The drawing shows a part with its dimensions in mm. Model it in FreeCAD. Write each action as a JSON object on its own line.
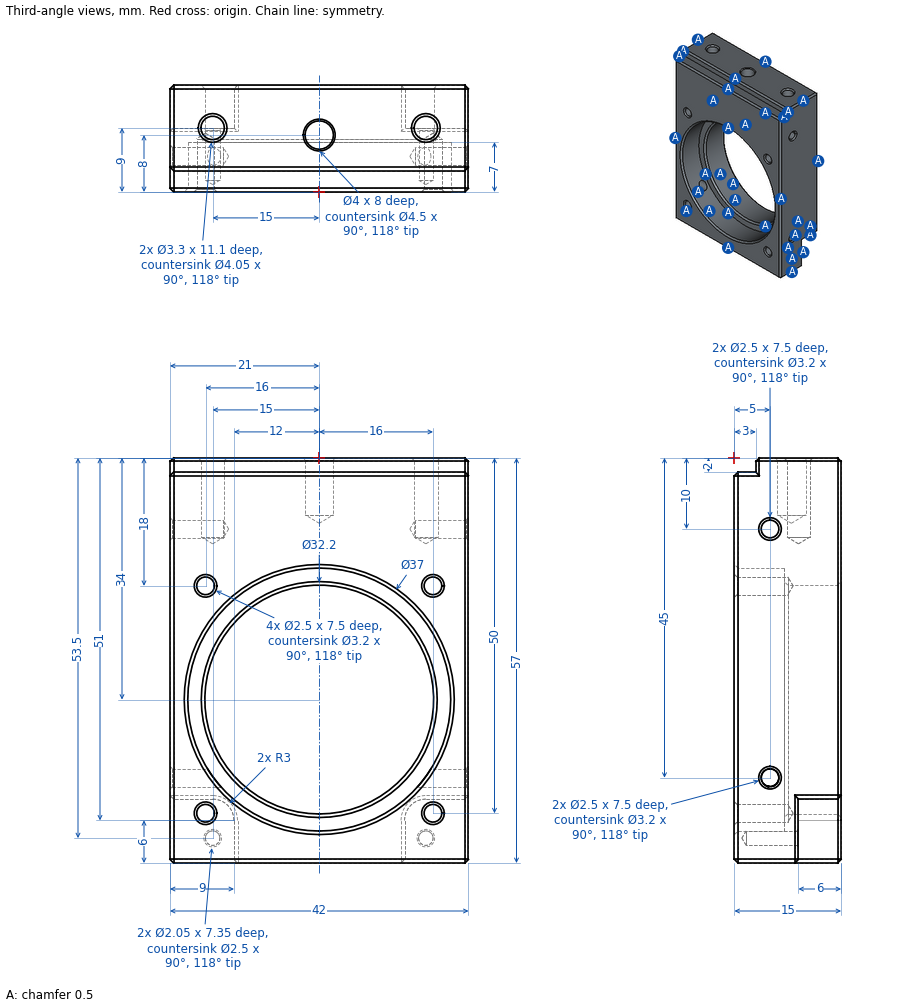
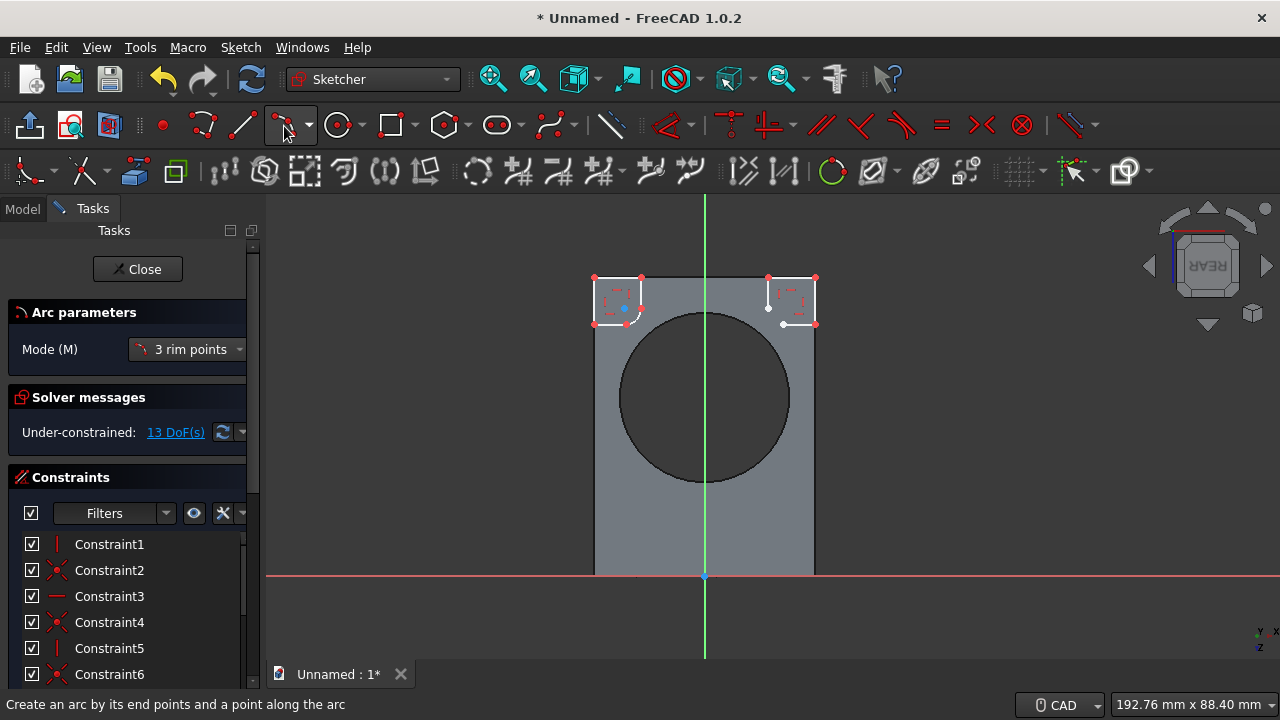
{"action": "left_click", "coordinate": [768, 309]}
{"action": "left_click", "coordinate": [783, 325]}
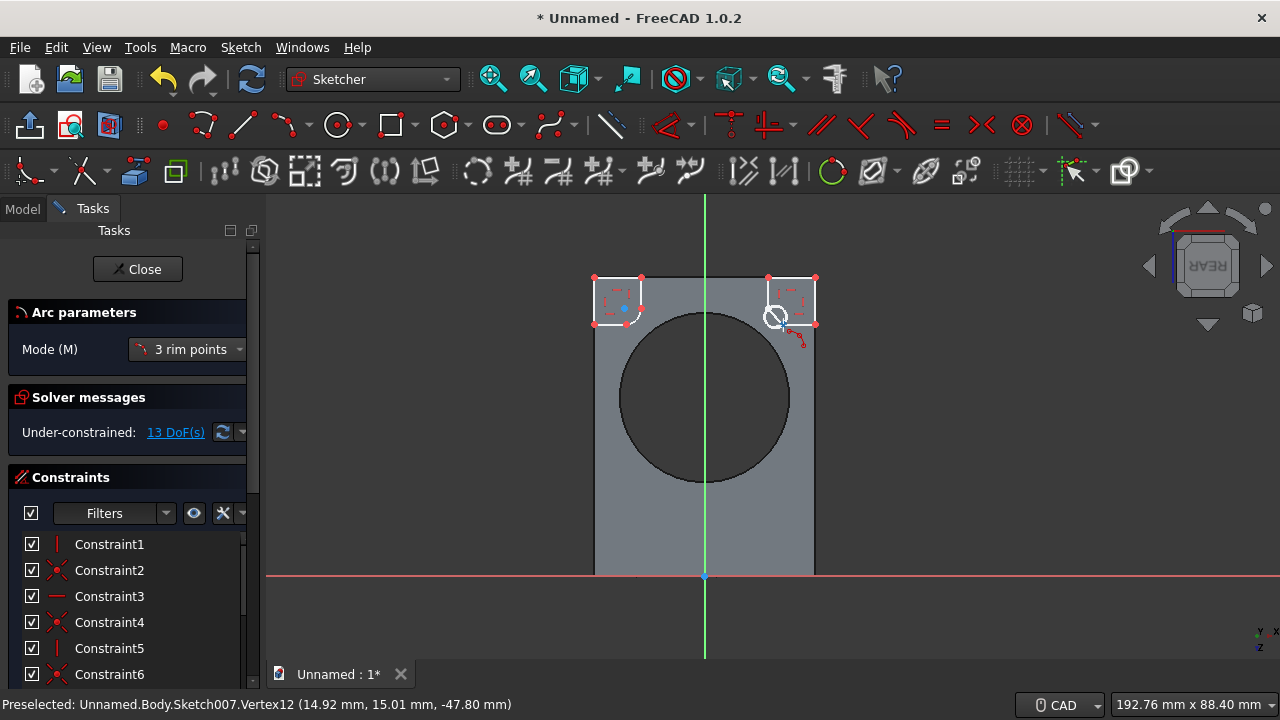
{"action": "scroll", "coordinate": [772, 319], "scroll_direction": "up", "scroll_amount": 7}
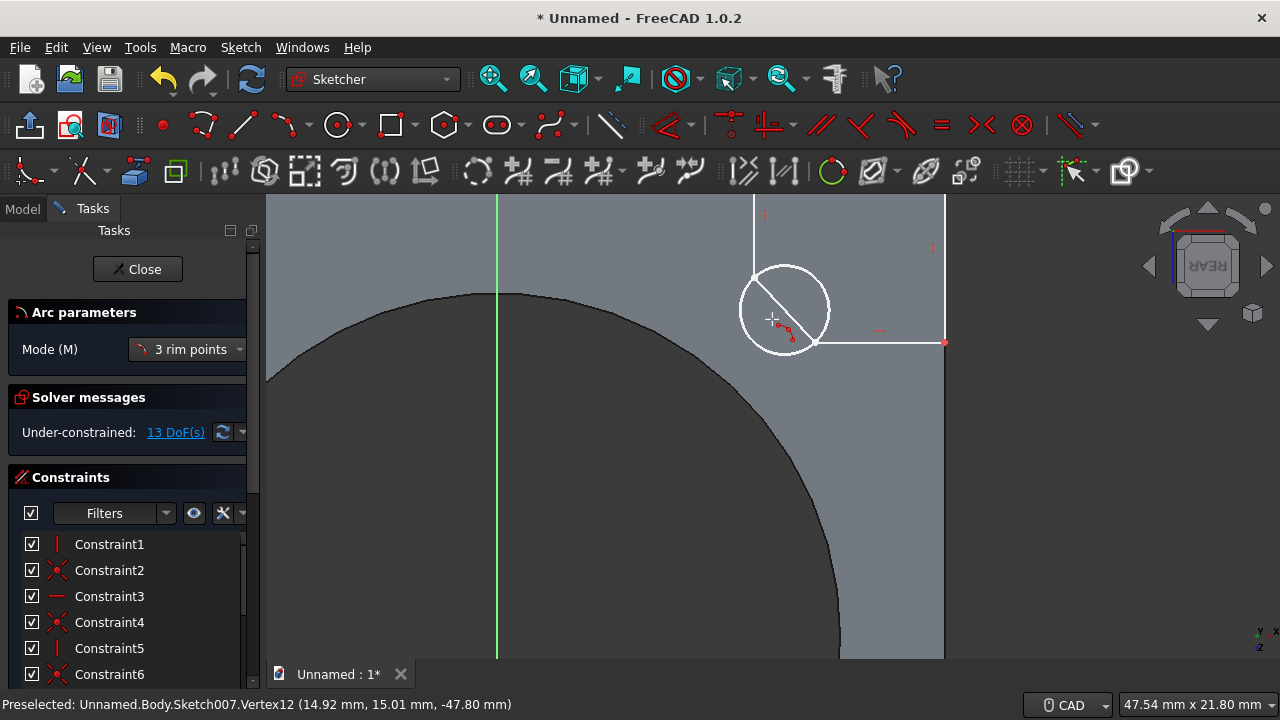
{"action": "left_click", "coordinate": [771, 319]}
{"action": "key", "text": "Escape"}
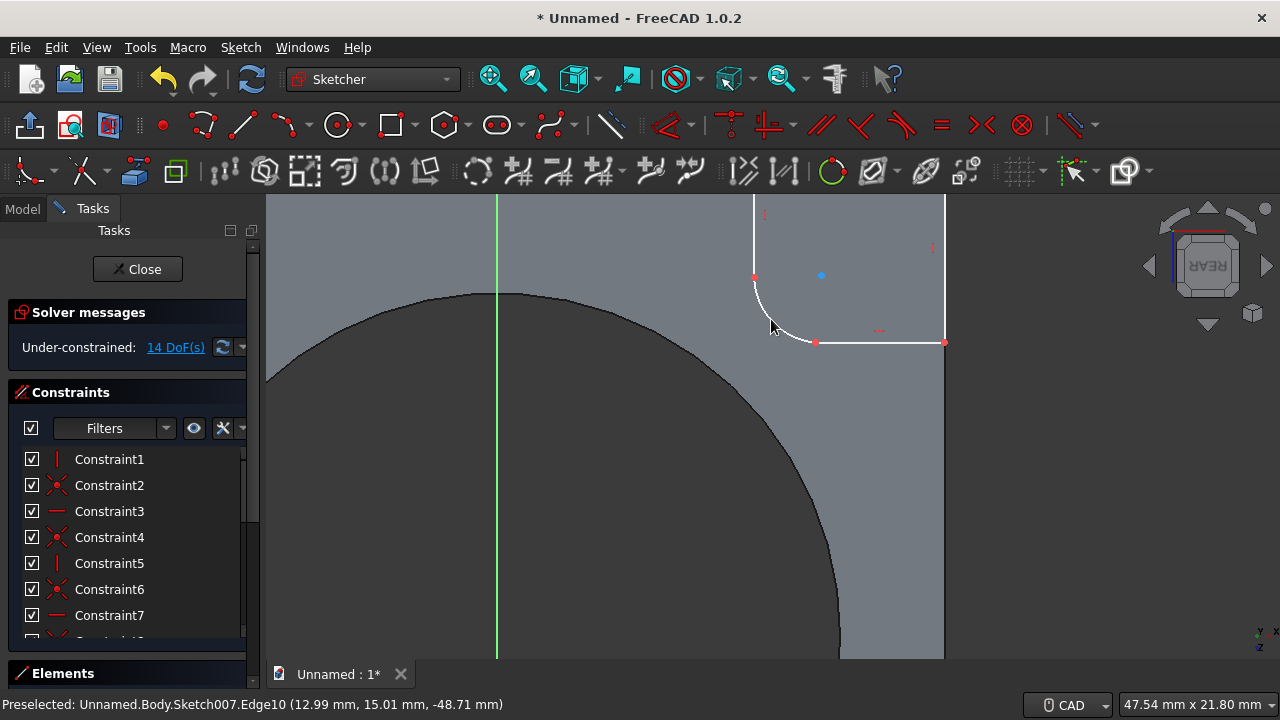
{"action": "scroll", "coordinate": [772, 319], "scroll_direction": "down", "scroll_amount": 7}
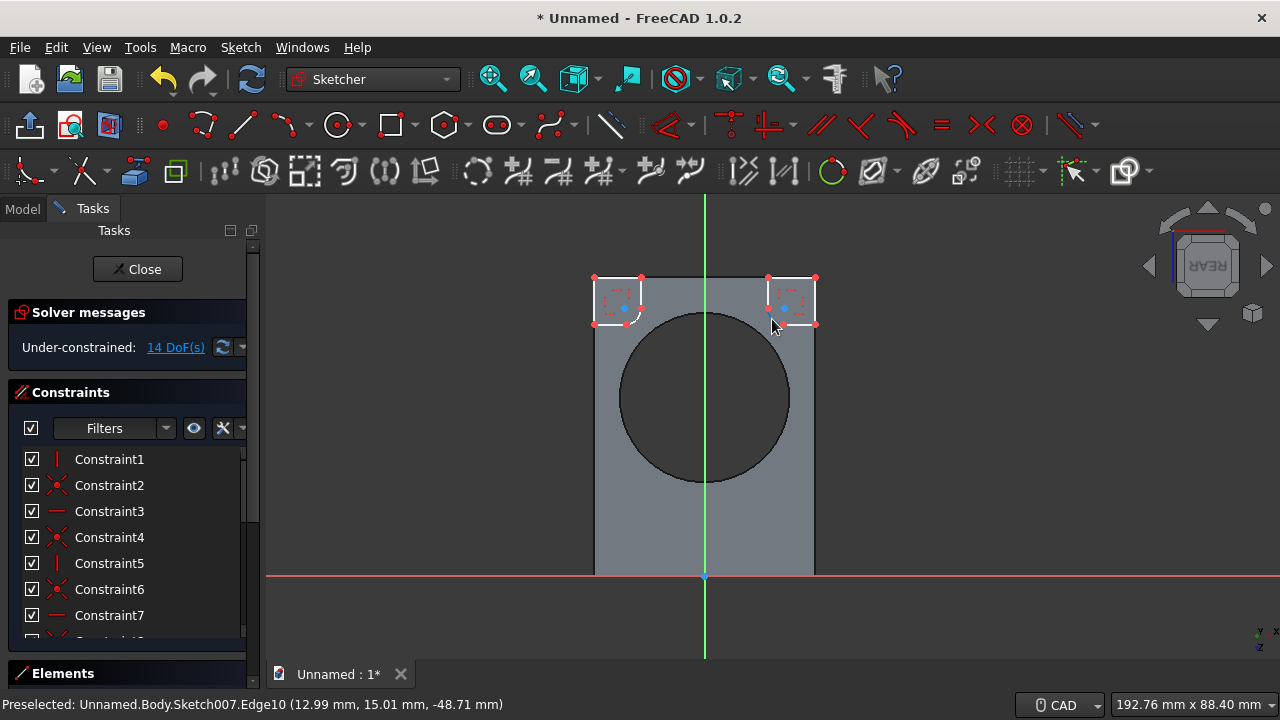
{"action": "scroll", "coordinate": [641, 300], "scroll_direction": "up", "scroll_amount": 2}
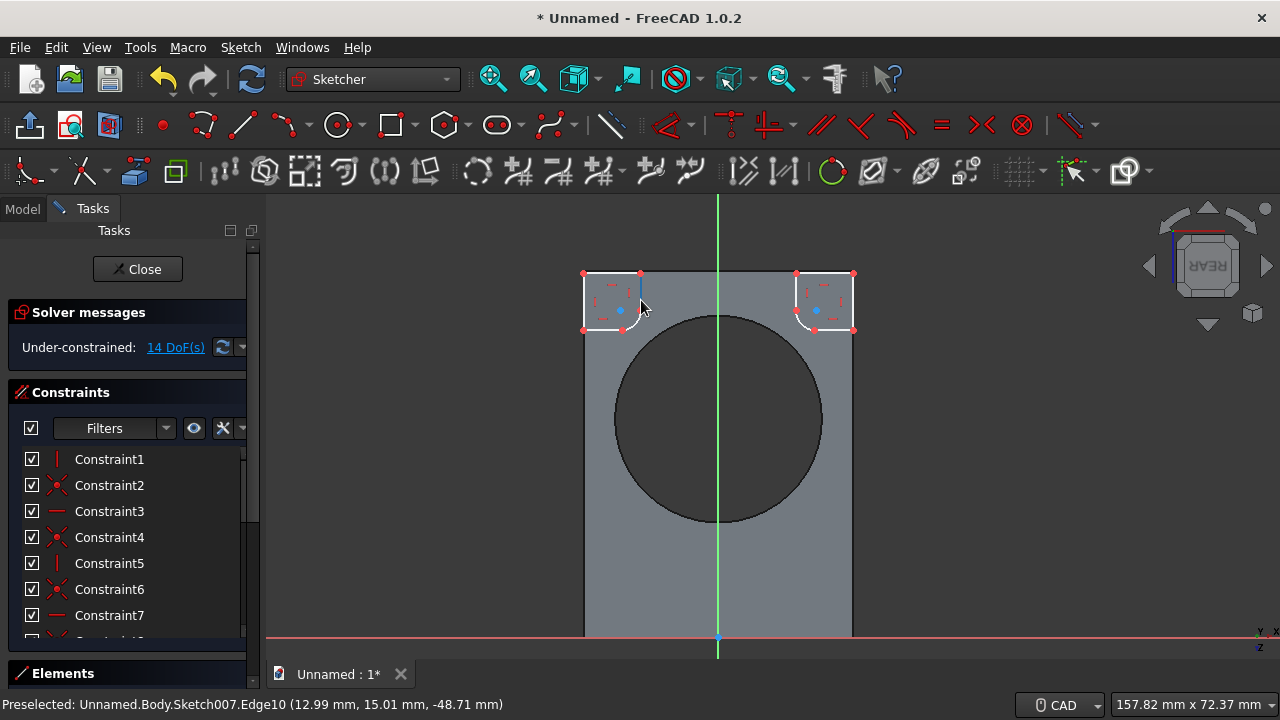
{"action": "left_click", "coordinate": [641, 299]}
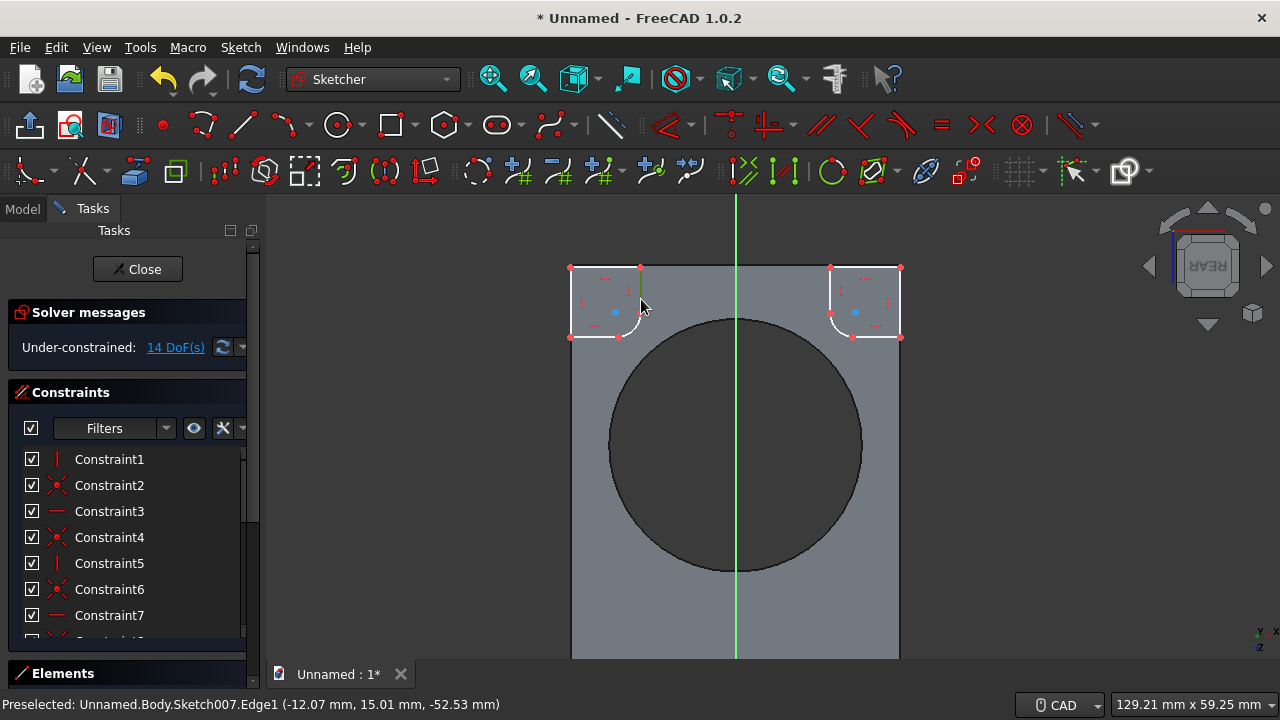
{"action": "scroll", "coordinate": [629, 334], "scroll_direction": "up", "scroll_amount": 2}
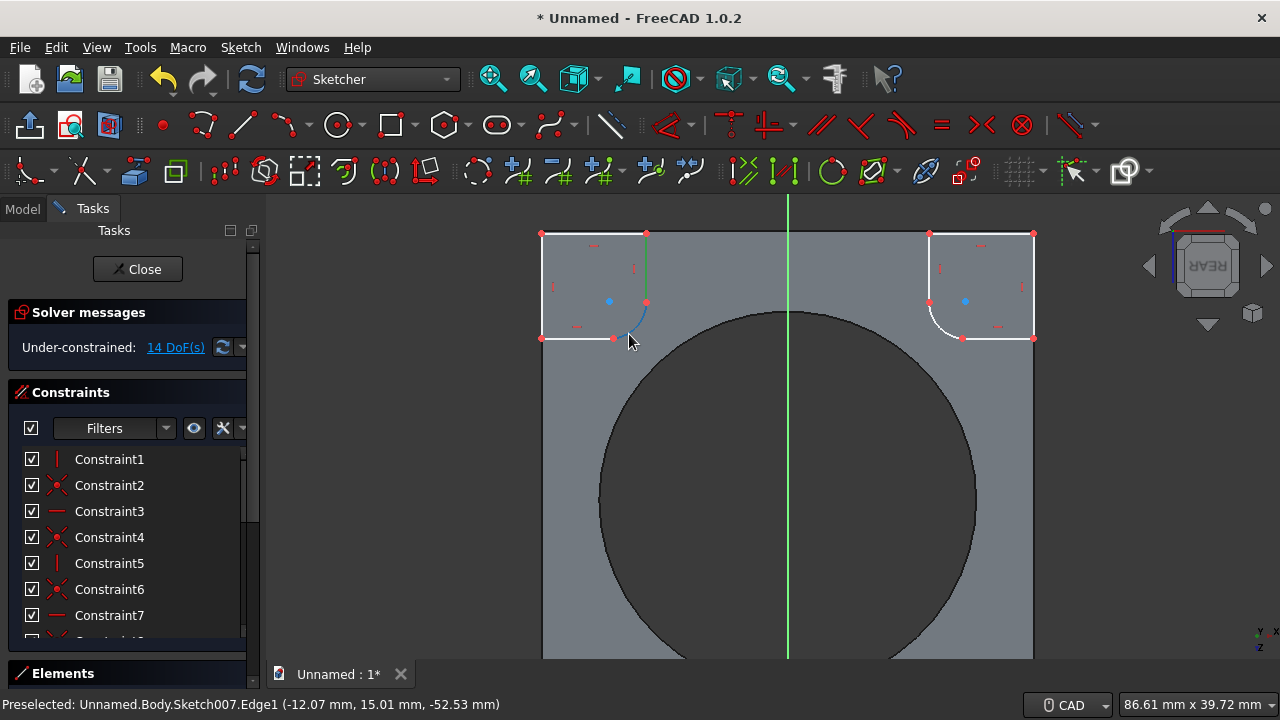
{"action": "left_click", "coordinate": [628, 334]}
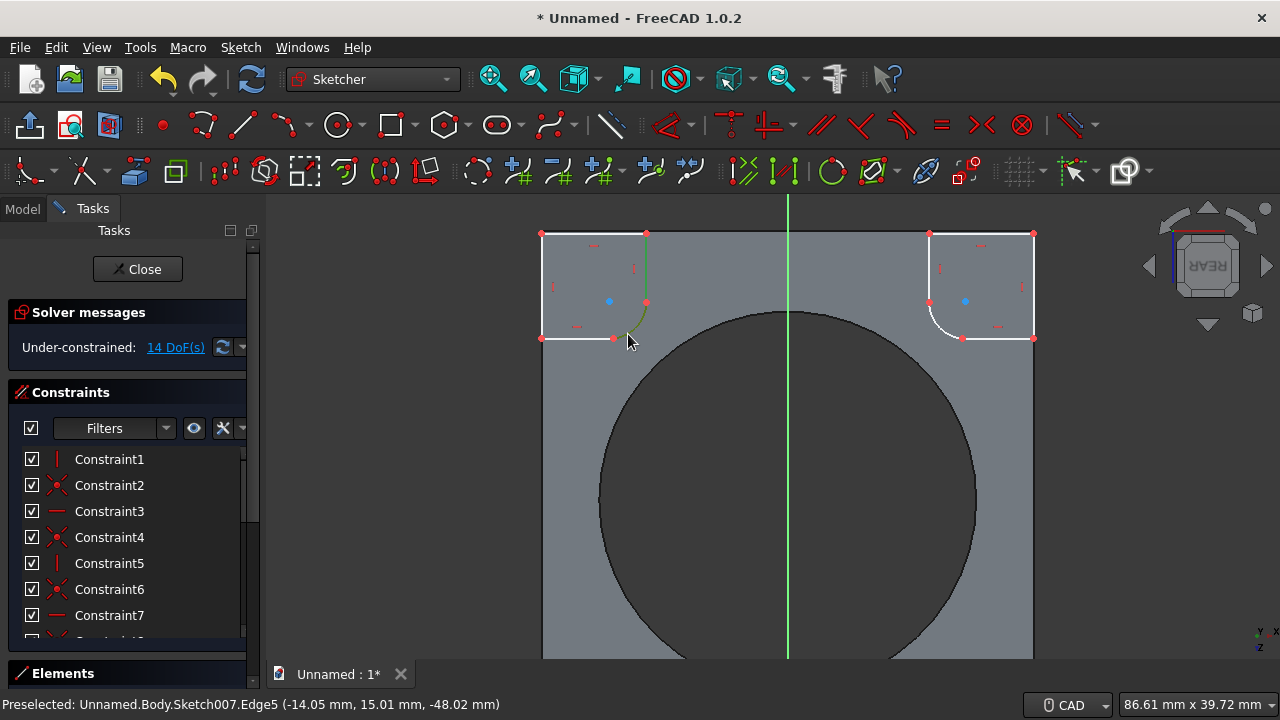
{"action": "key", "text": "t"}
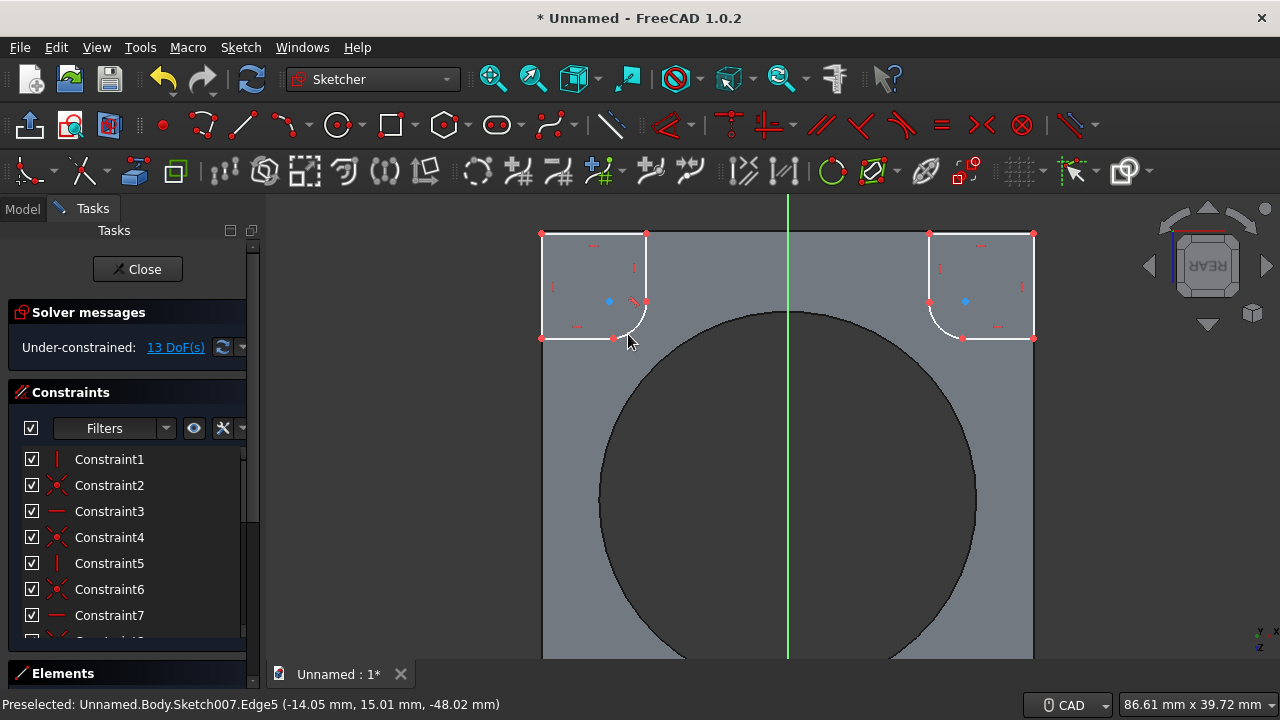
{"action": "left_click", "coordinate": [563, 339]}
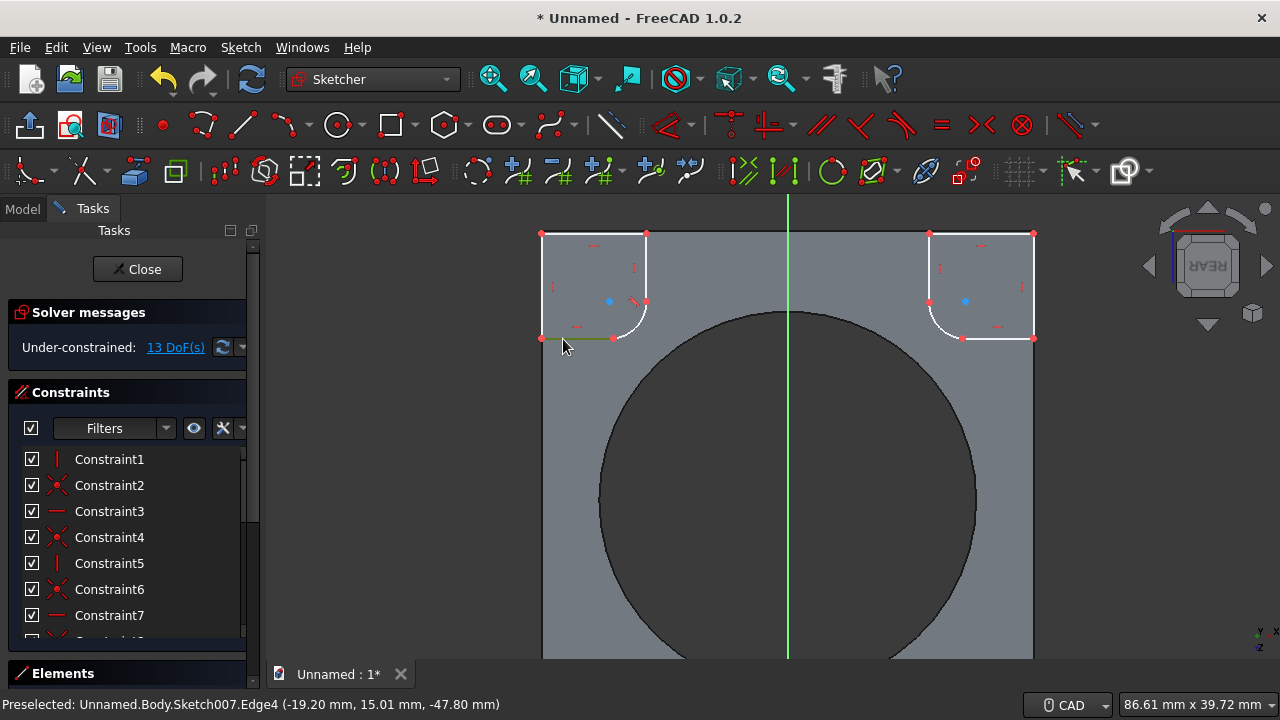
{"action": "left_click", "coordinate": [628, 333]}